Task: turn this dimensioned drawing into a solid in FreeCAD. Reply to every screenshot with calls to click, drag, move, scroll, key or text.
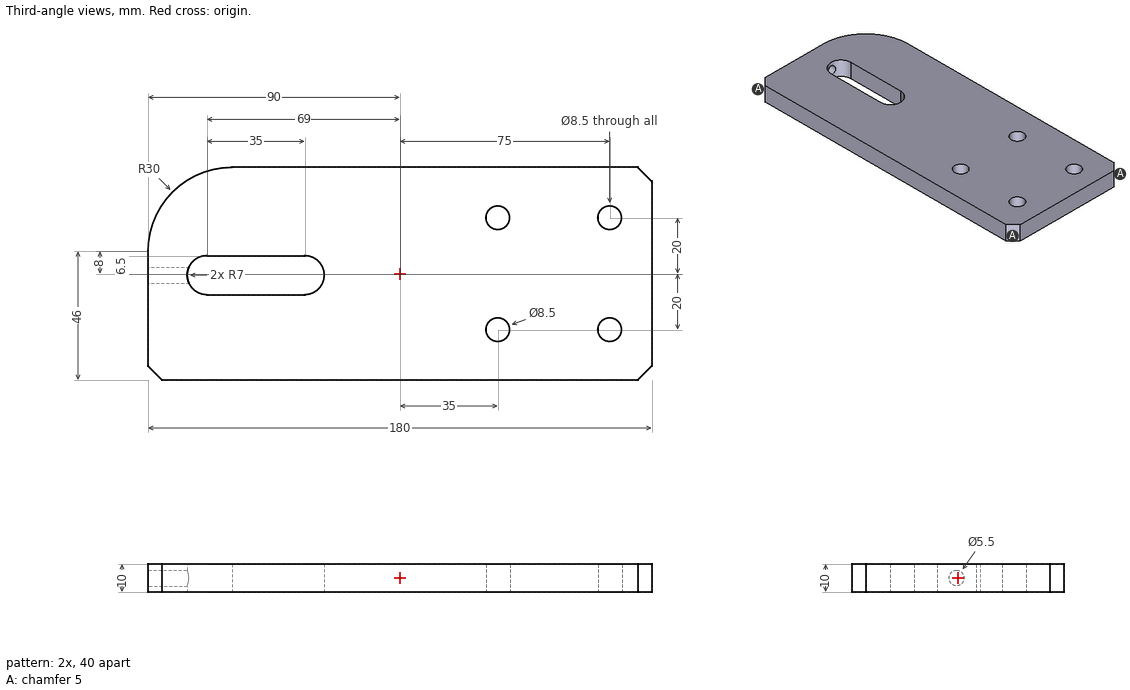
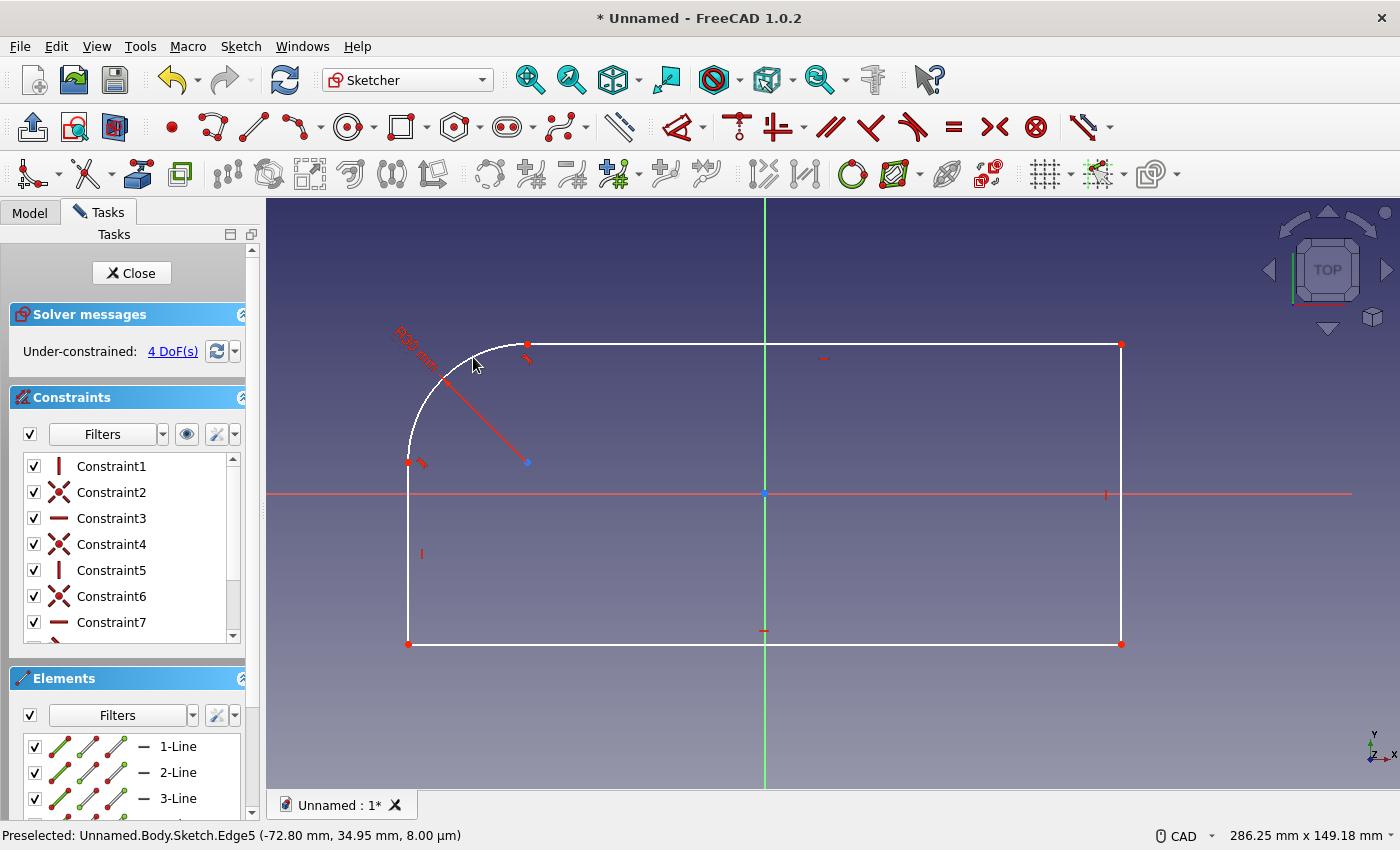
click(408, 517)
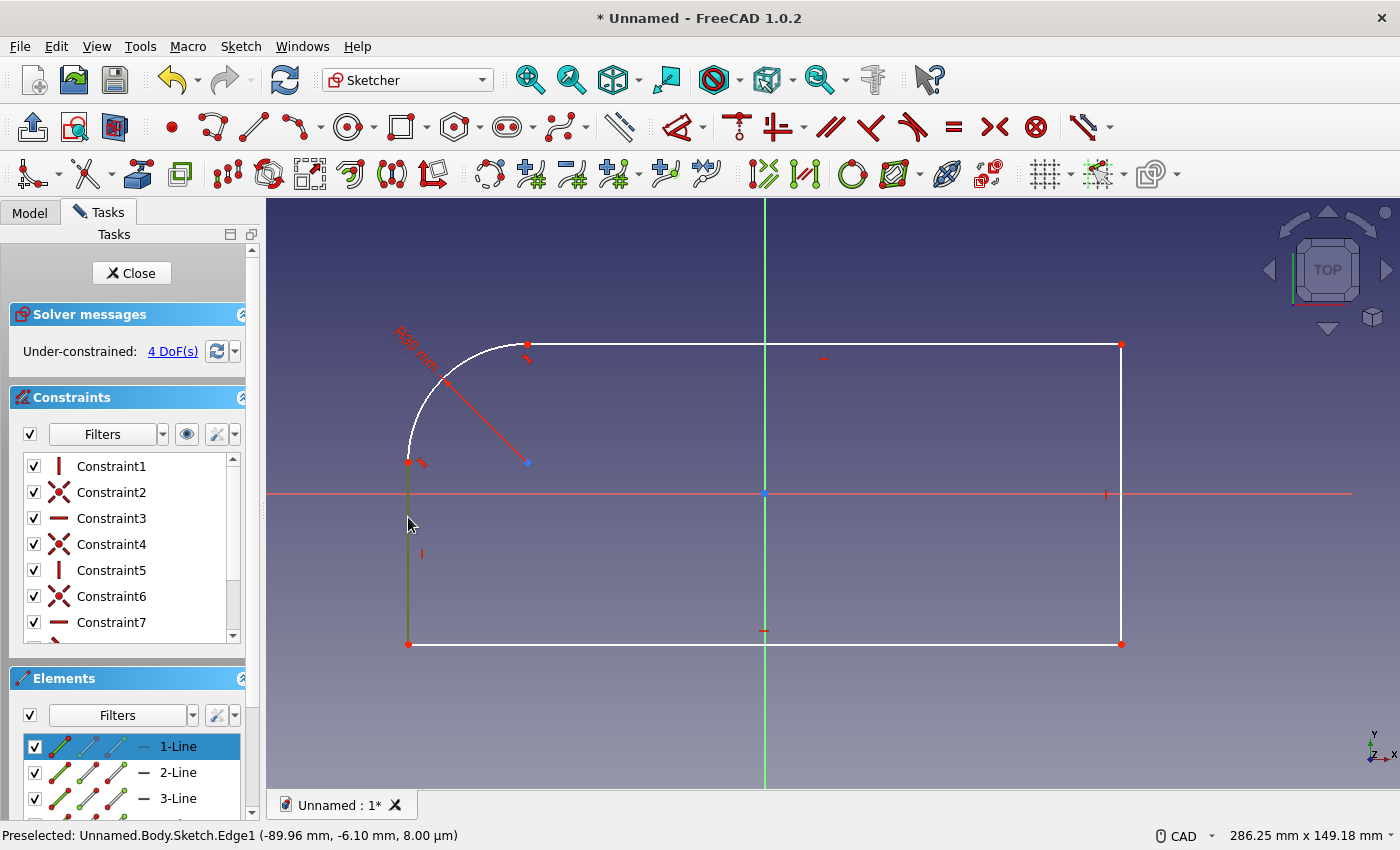
click(702, 128)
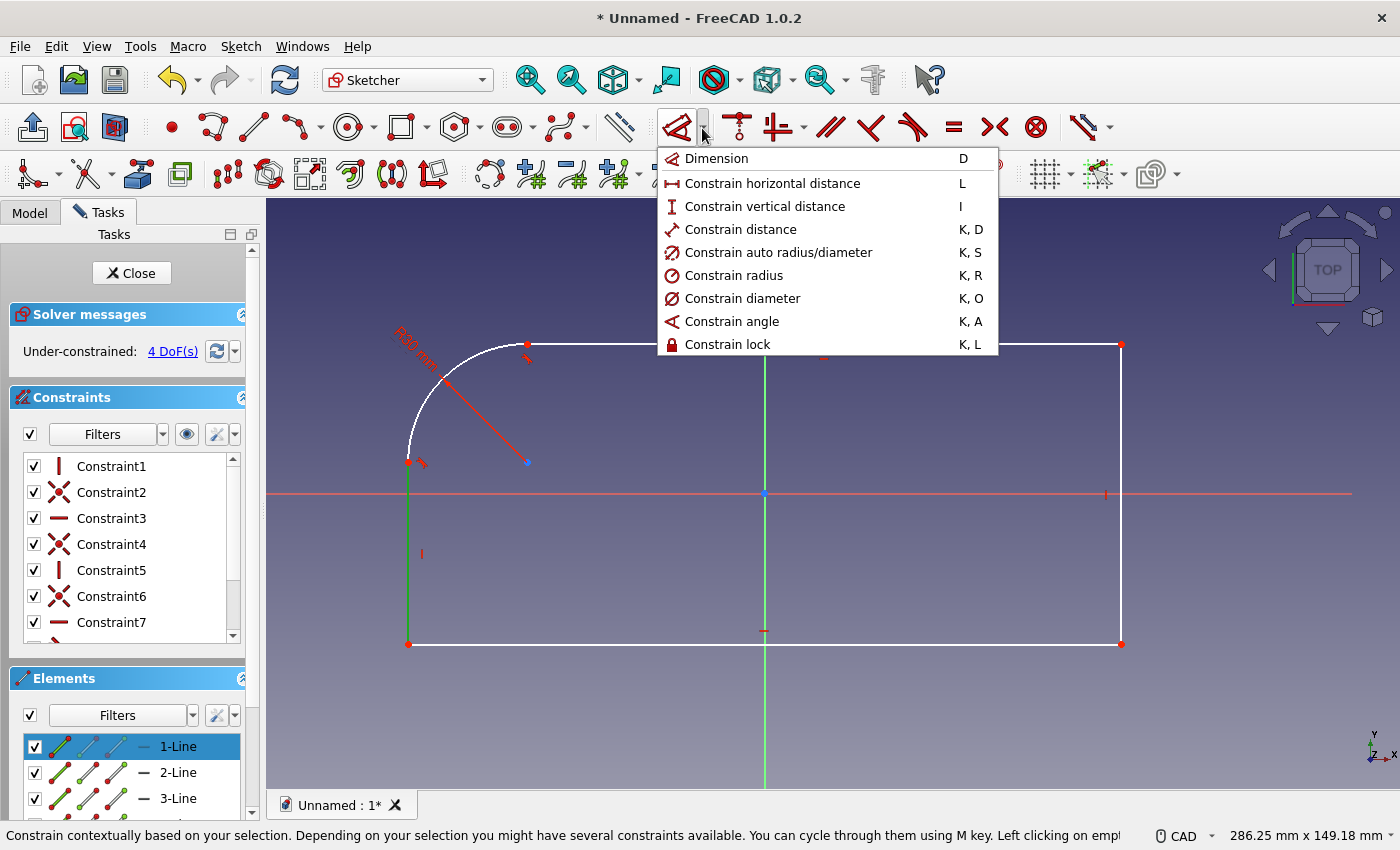
click(828, 206)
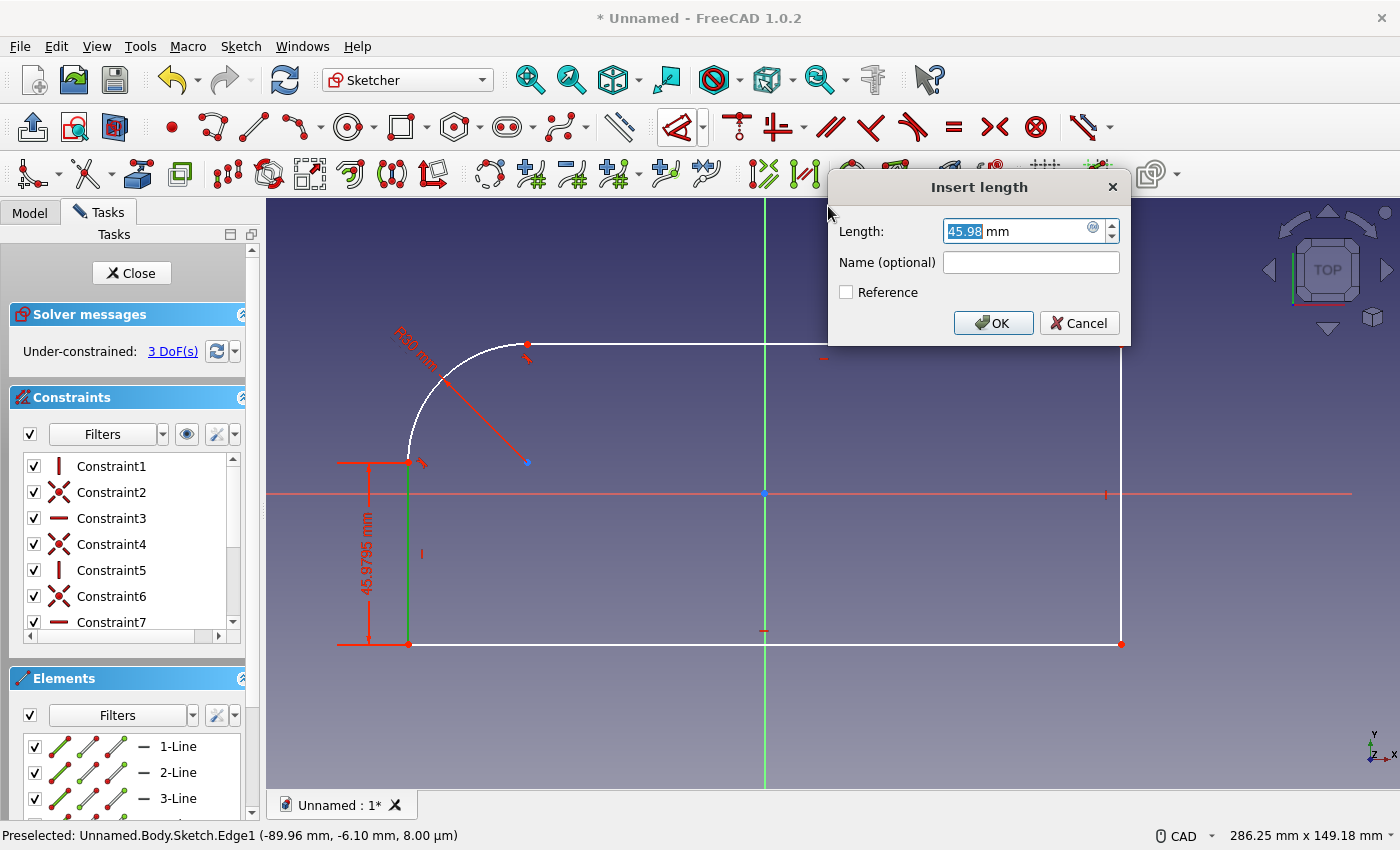
text(46)
key(Return)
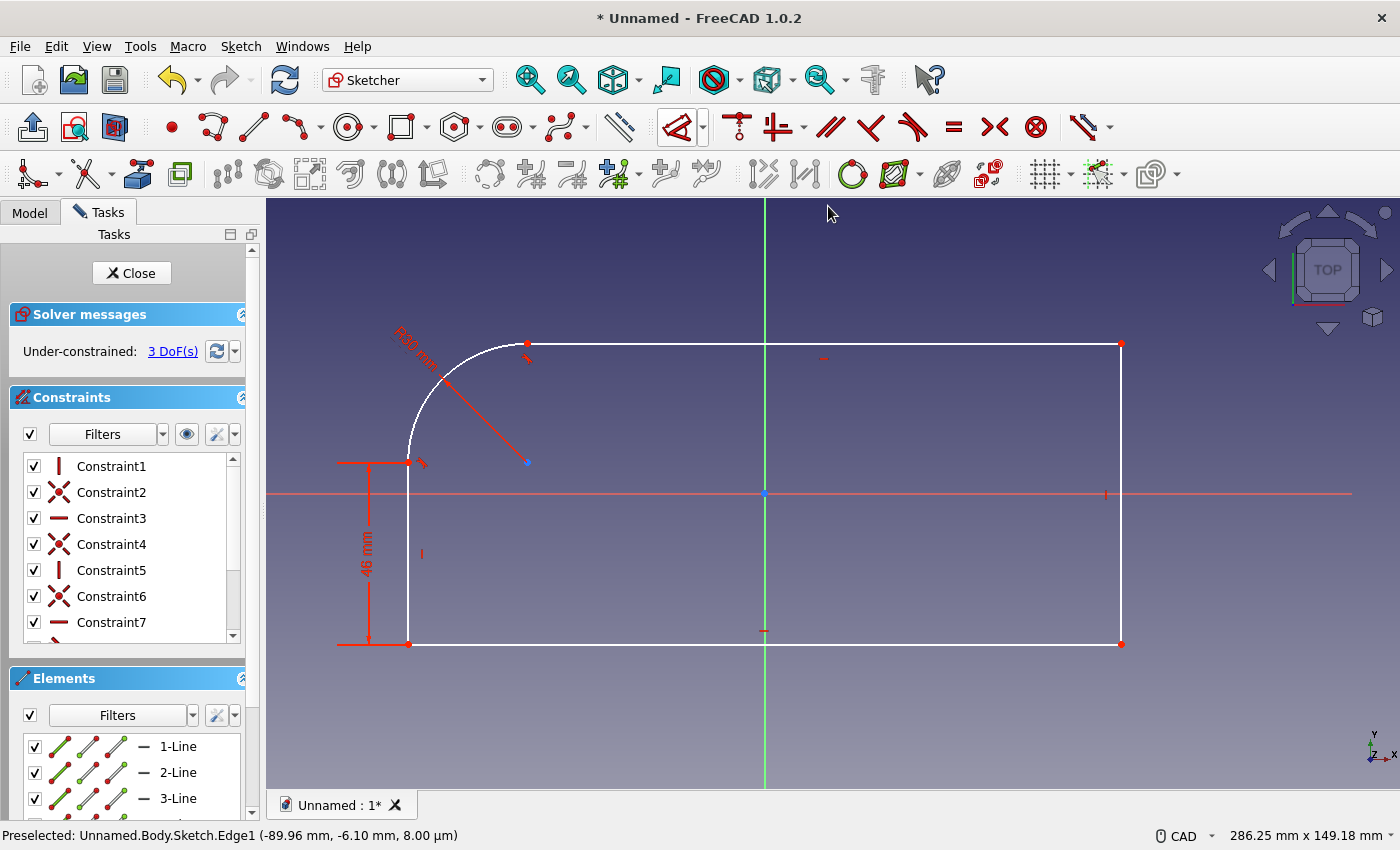
scroll(408, 463, up, 2)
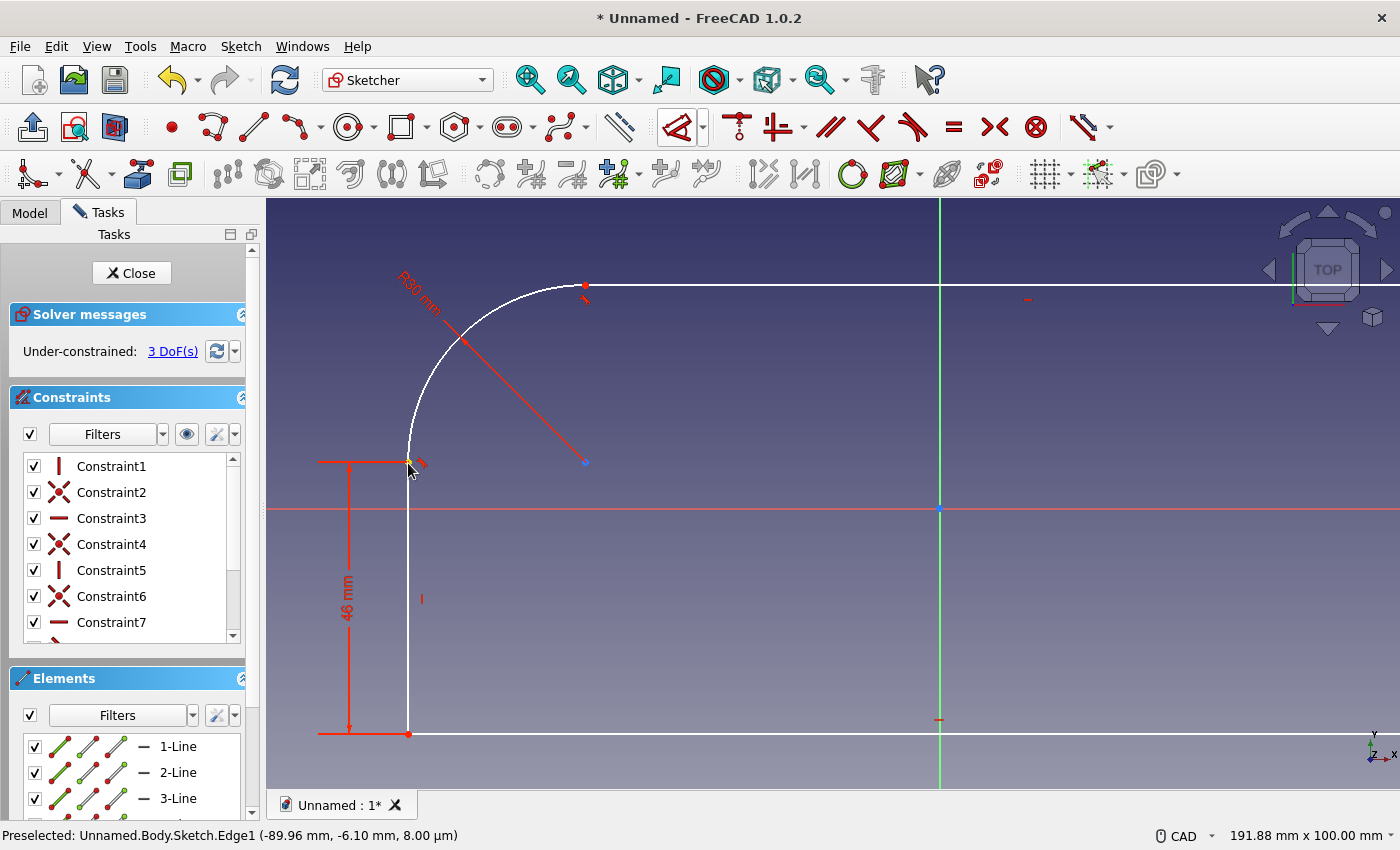
click(408, 462)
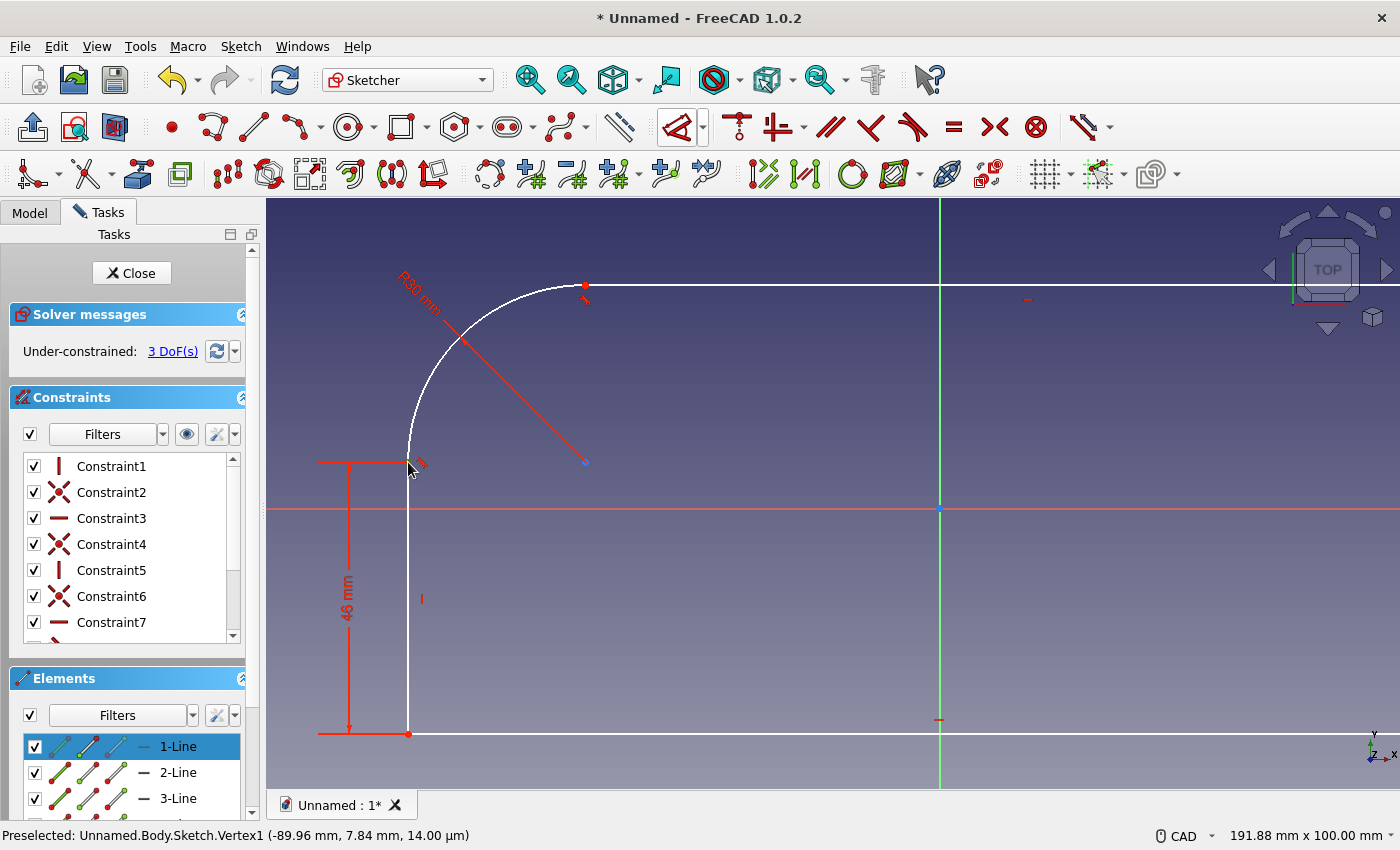
key(i)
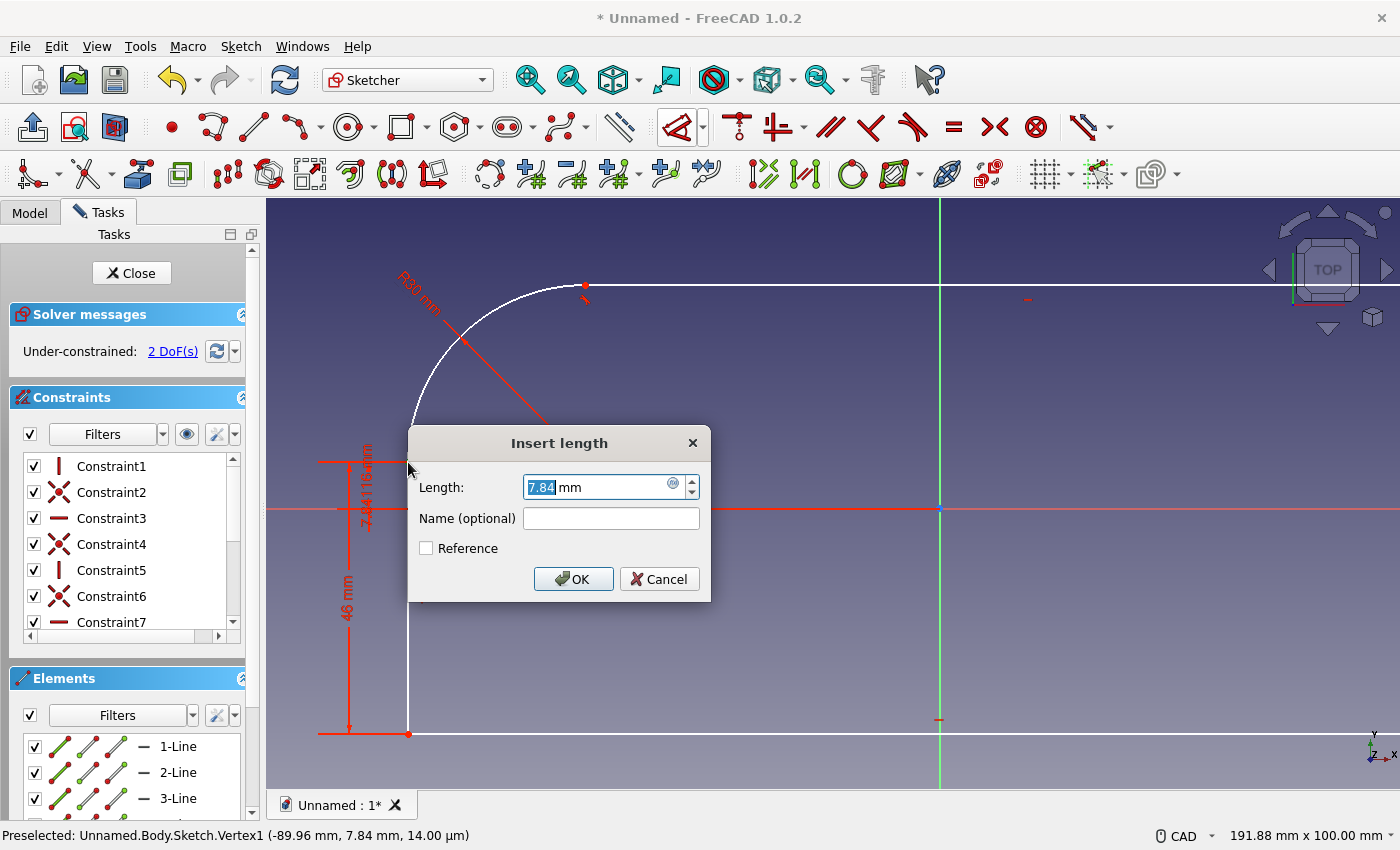
text(8)
key(Return)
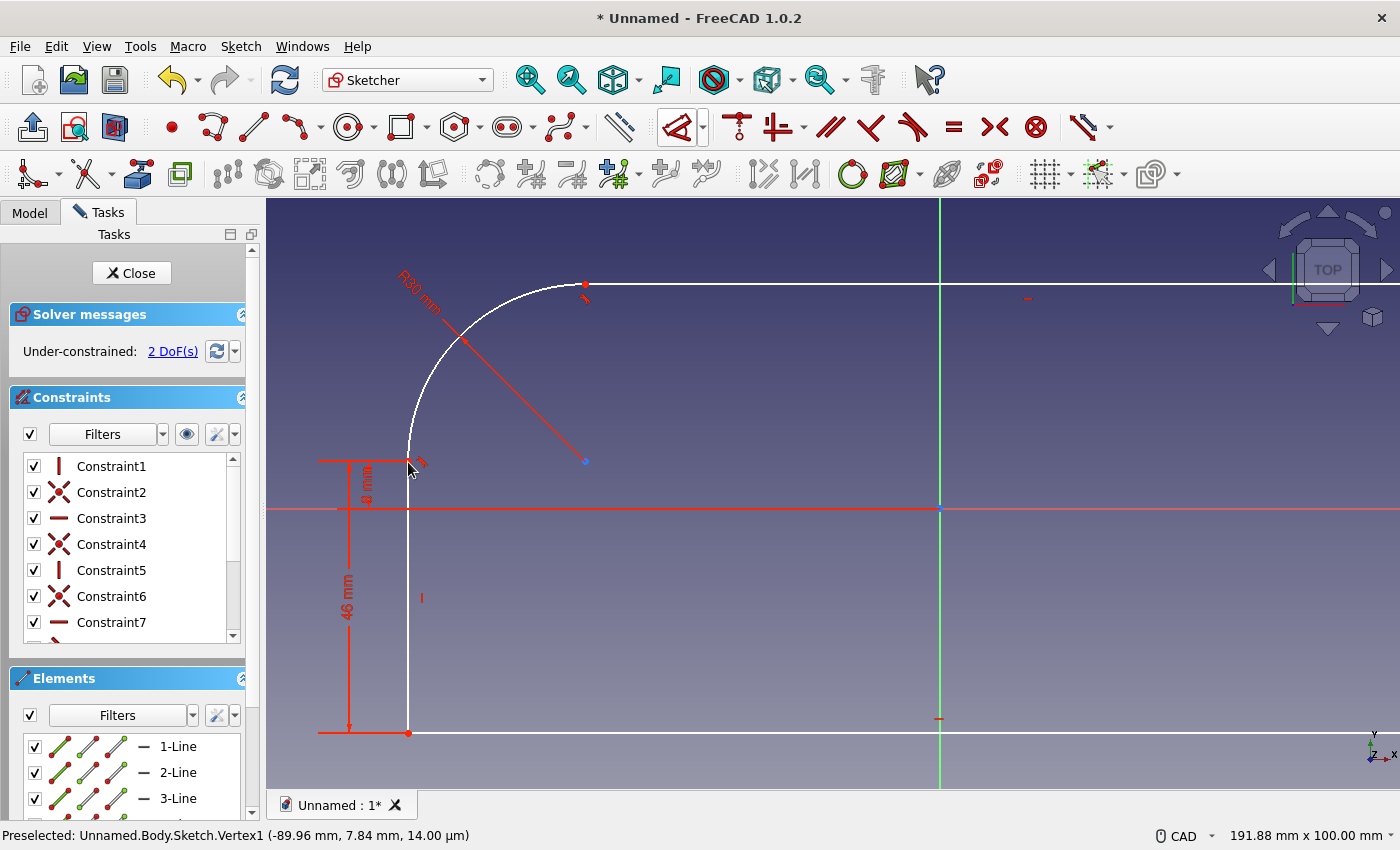
click(727, 733)